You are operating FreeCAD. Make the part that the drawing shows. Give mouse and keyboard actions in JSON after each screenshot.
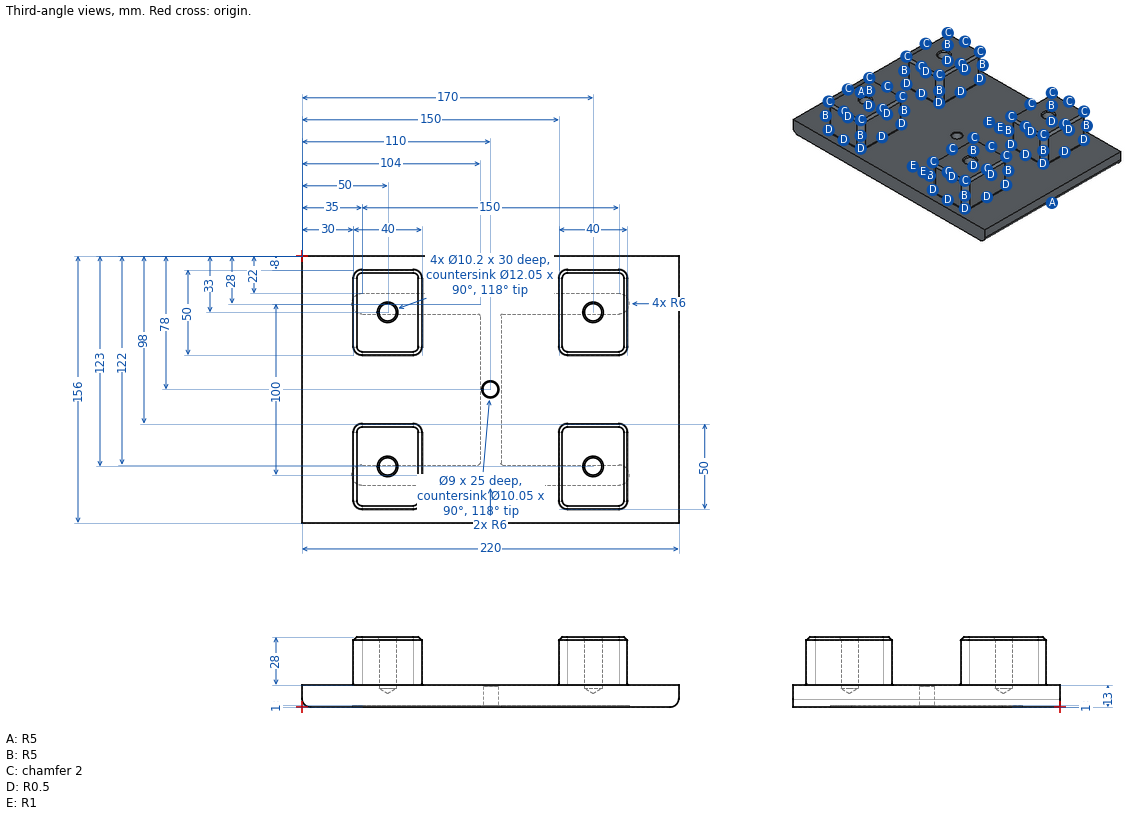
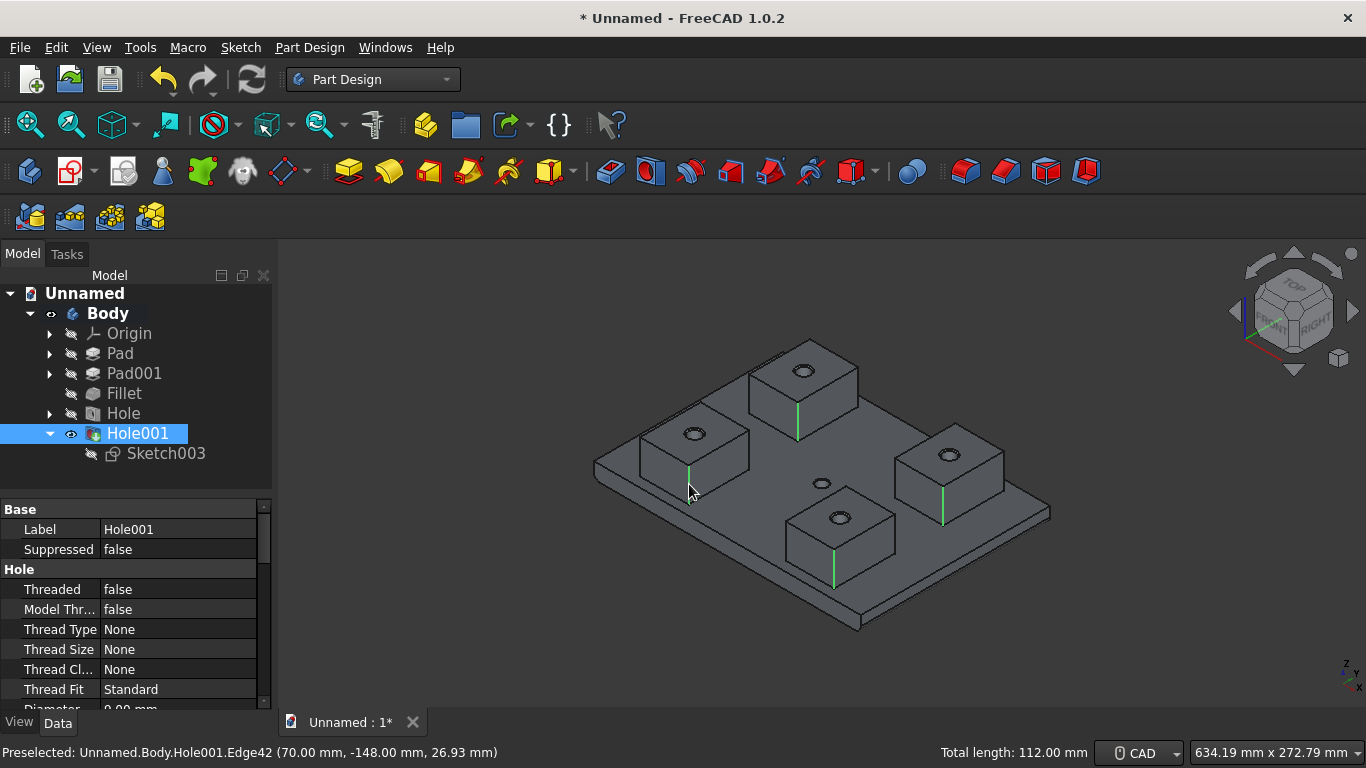
{"action": "key", "text": "1"}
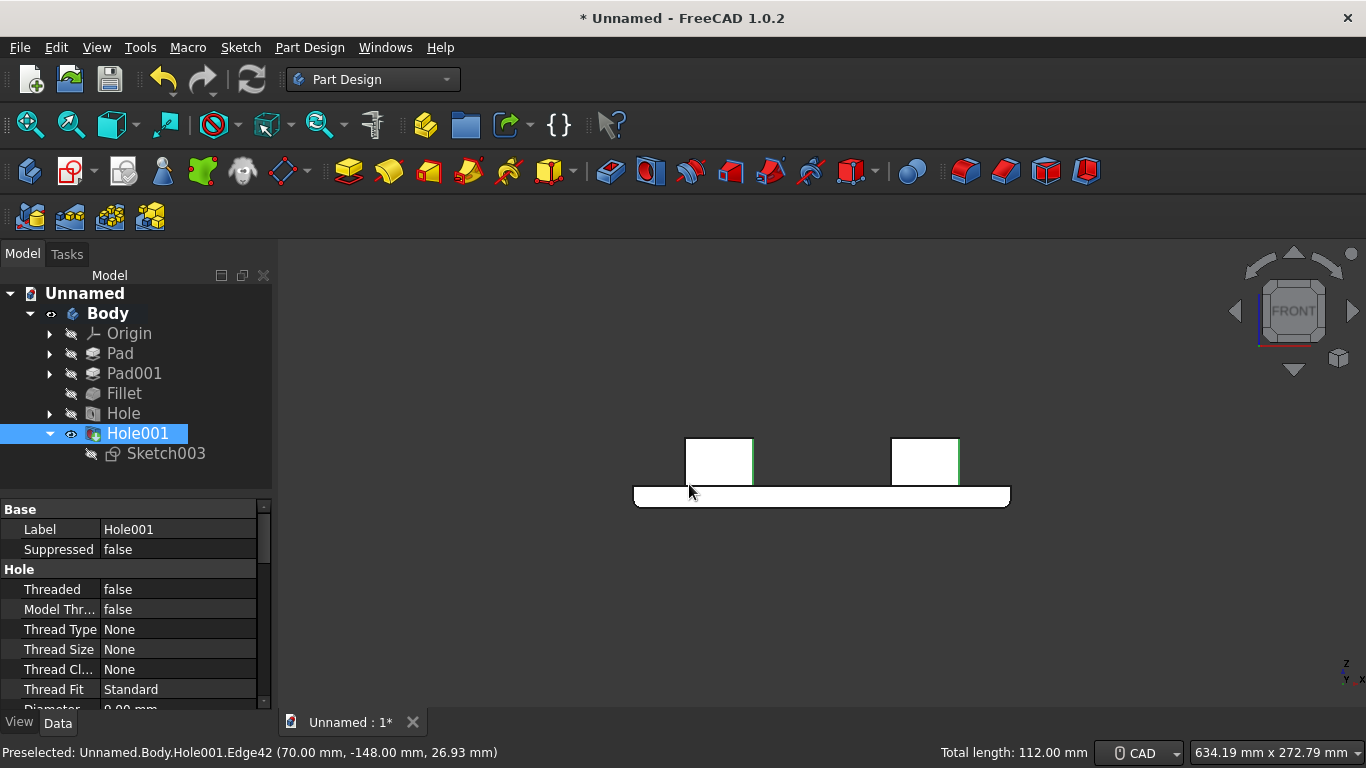
{"action": "left_click", "coordinate": [32, 126]}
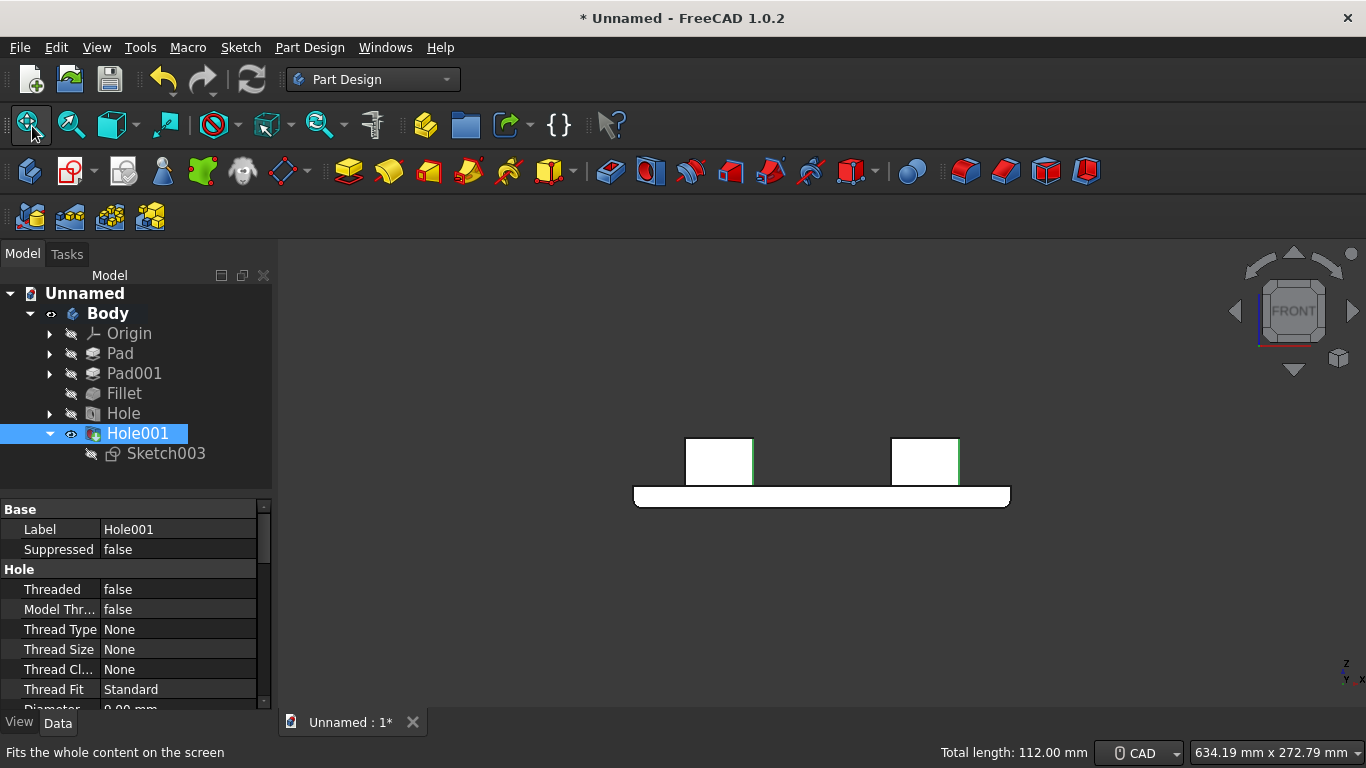
{"action": "left_click", "coordinate": [891, 461], "text": "ctrl"}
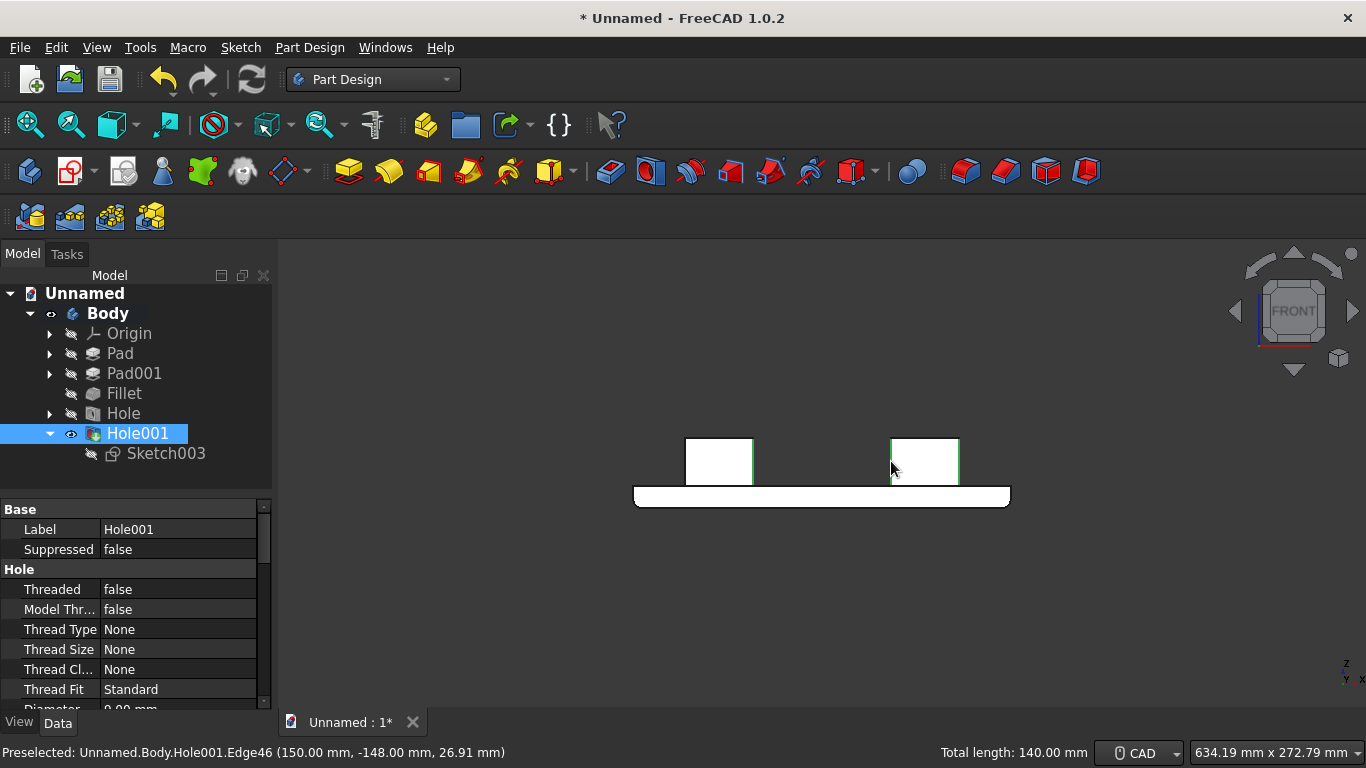
{"action": "left_click", "coordinate": [685, 461], "text": "ctrl"}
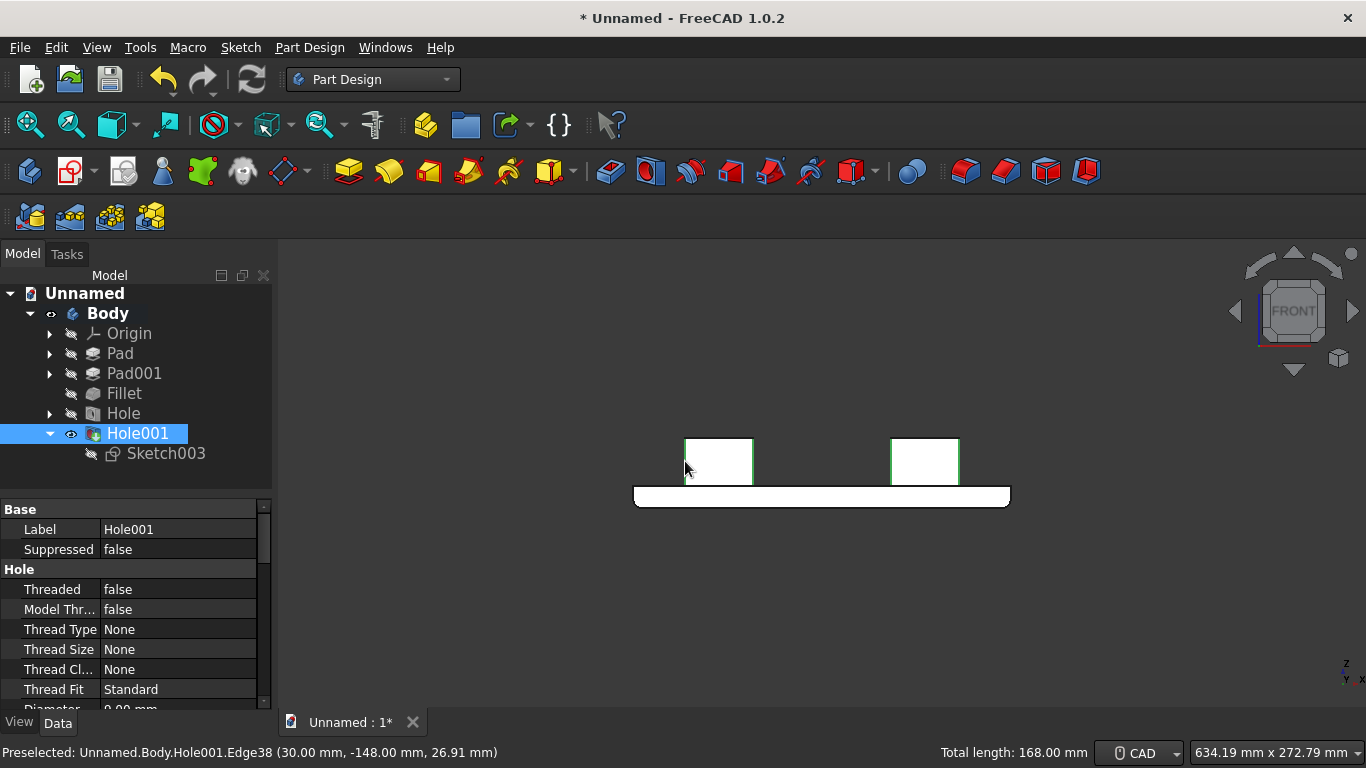
{"action": "key", "text": "3"}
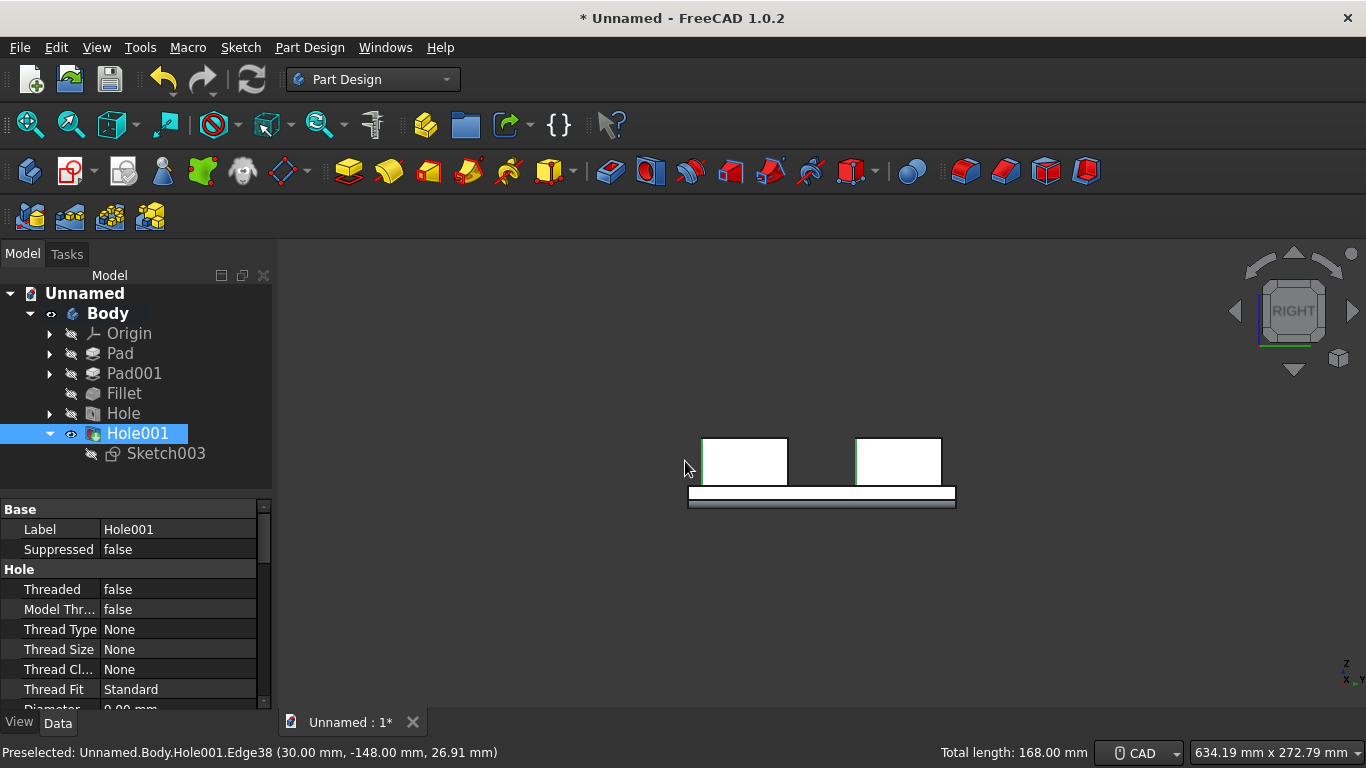
{"action": "key", "text": "v f"}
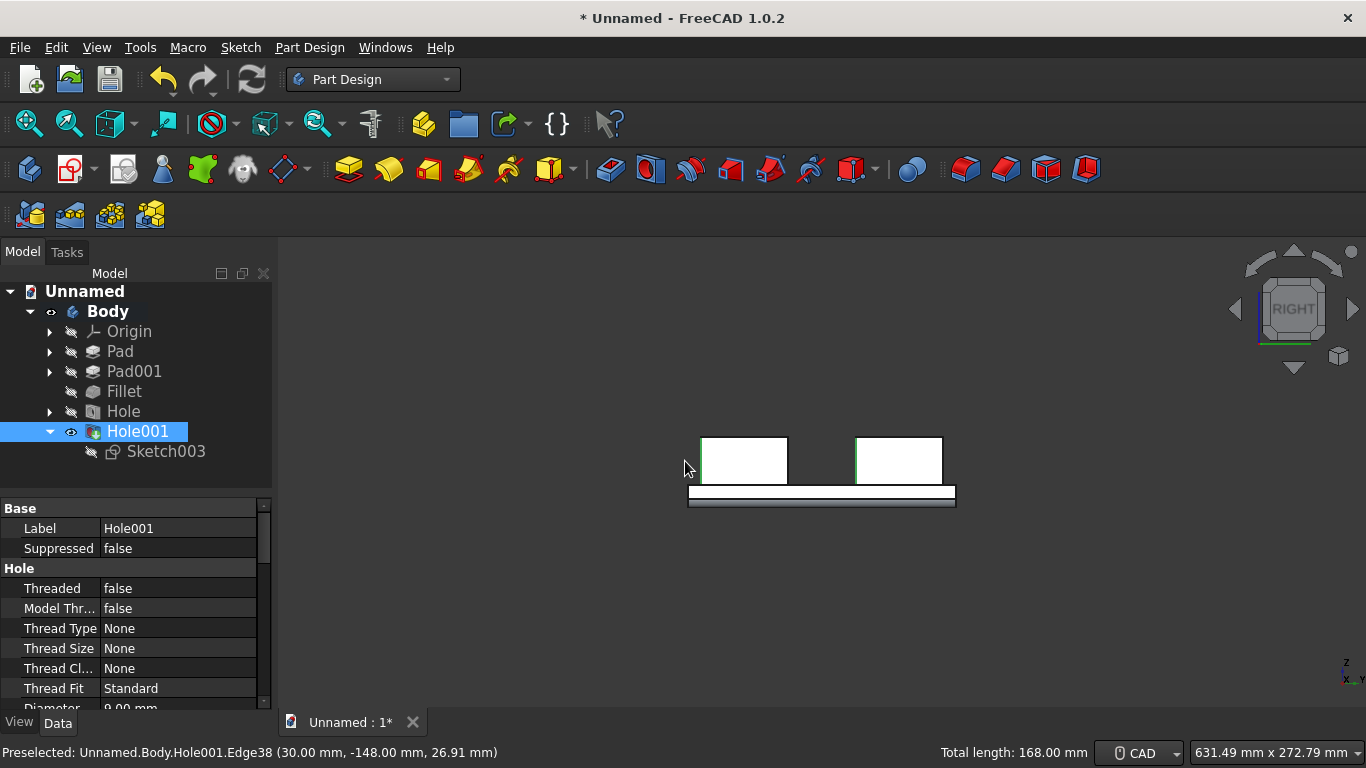
{"action": "left_click", "coordinate": [943, 460], "text": "ctrl"}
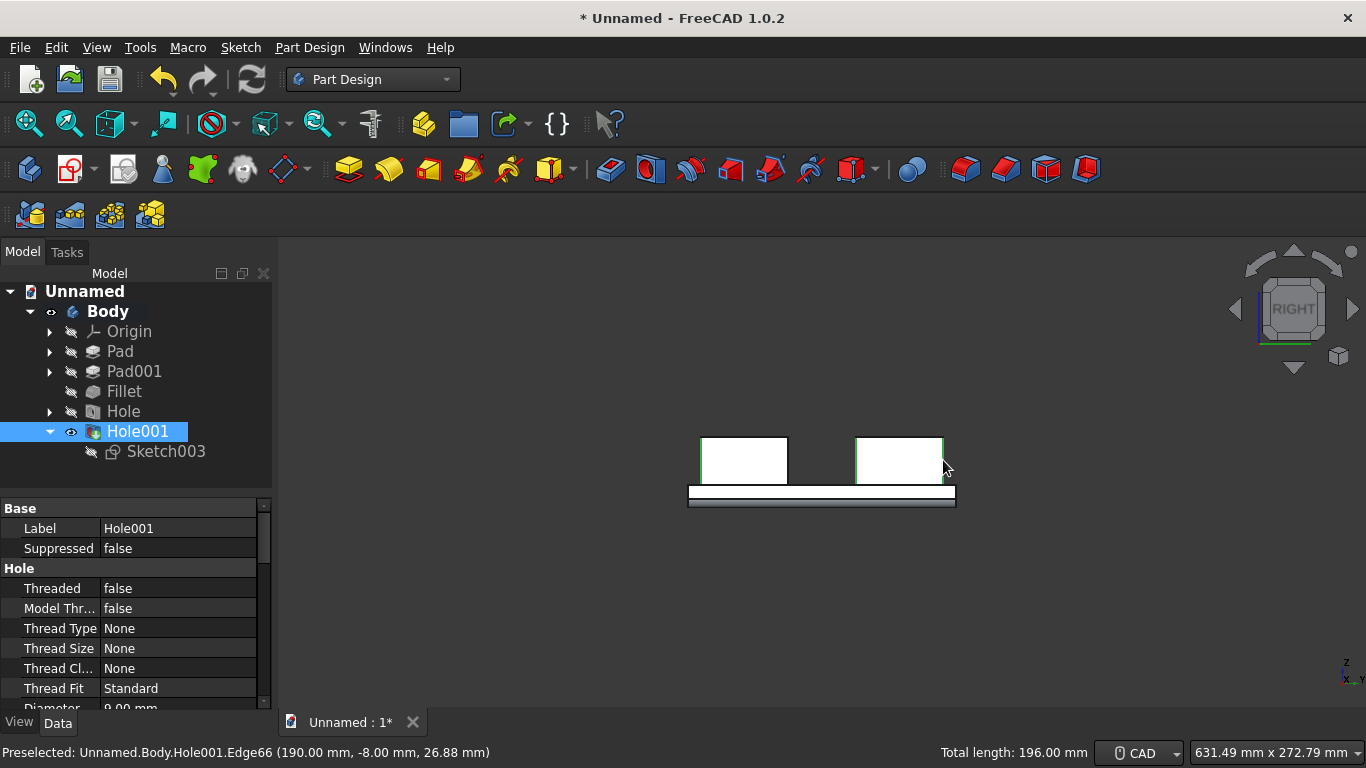
{"action": "left_click", "coordinate": [788, 460], "text": "ctrl"}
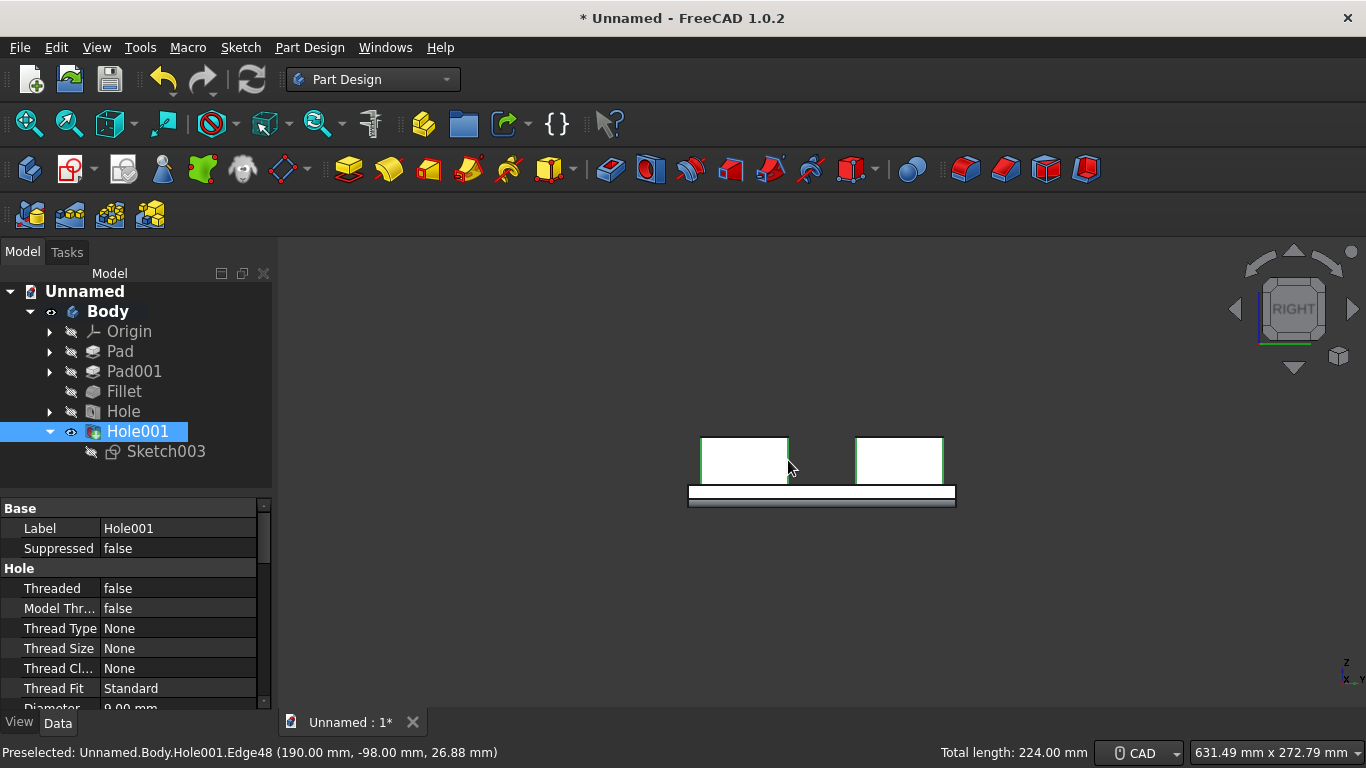
{"action": "key", "text": "5"}